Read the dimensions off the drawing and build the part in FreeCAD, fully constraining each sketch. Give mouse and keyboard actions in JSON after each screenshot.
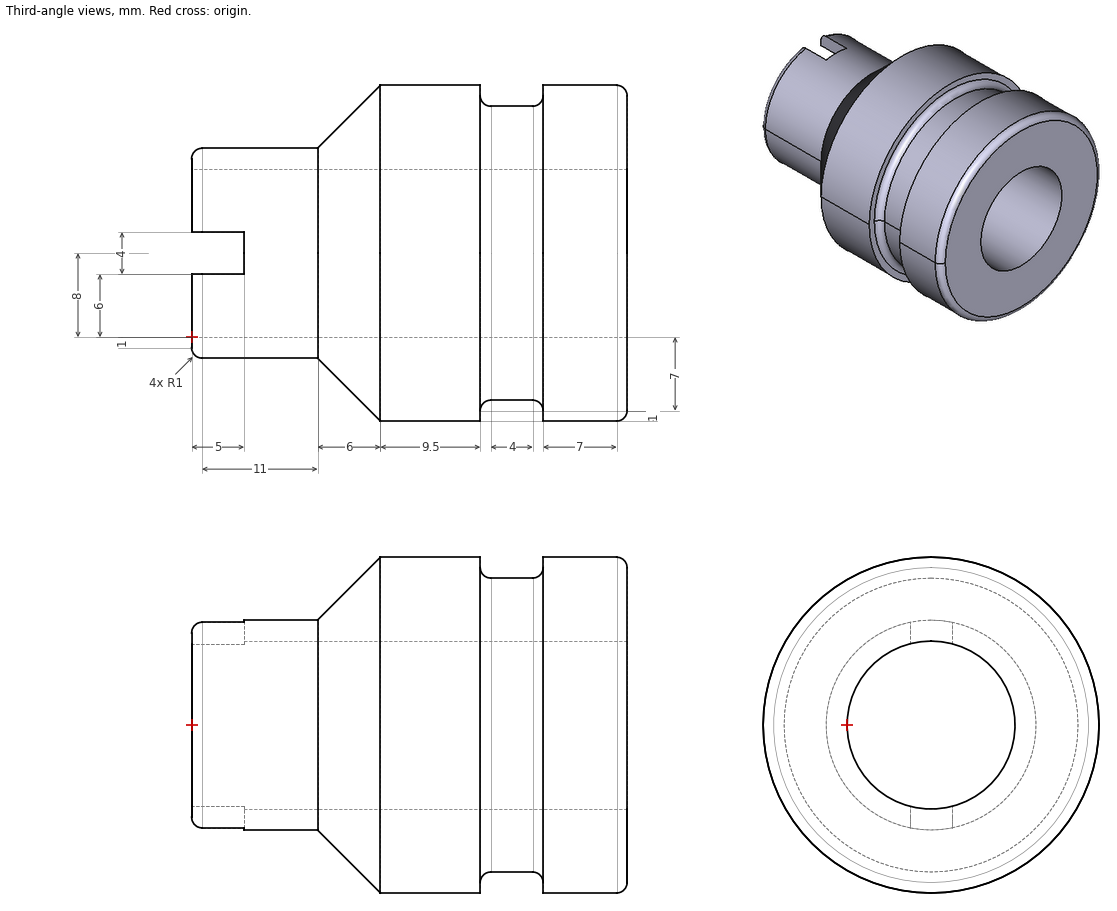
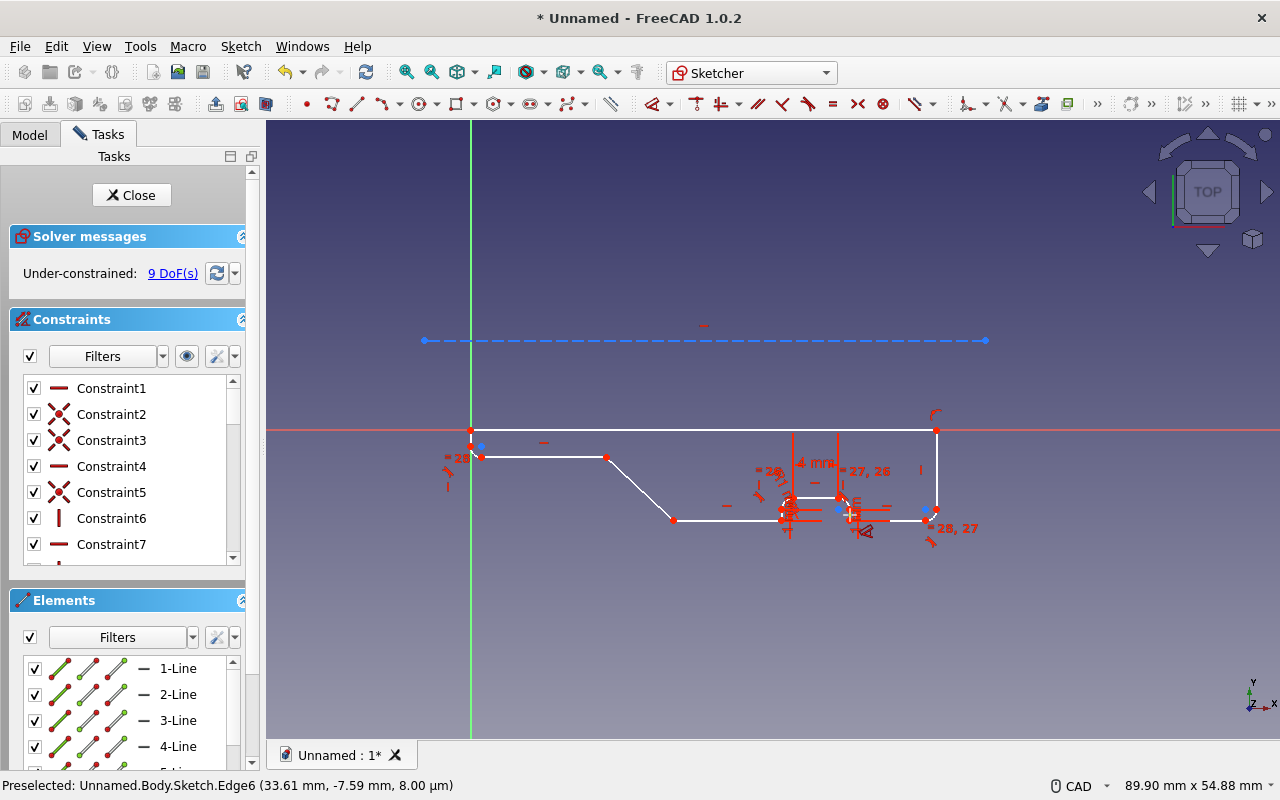
{"action": "left_click", "coordinate": [872, 521]}
{"action": "left_click", "coordinate": [888, 555]}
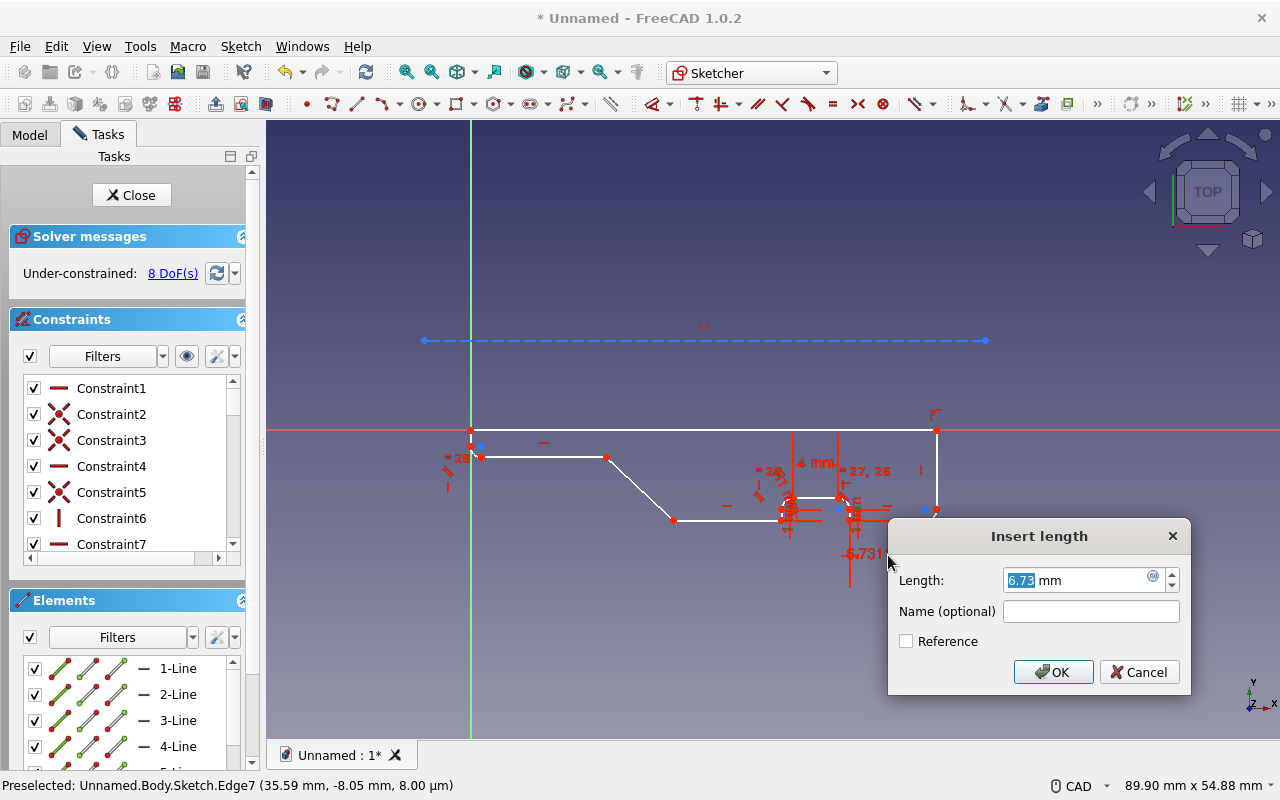
{"action": "type", "text": "7"}
{"action": "key", "text": "Return"}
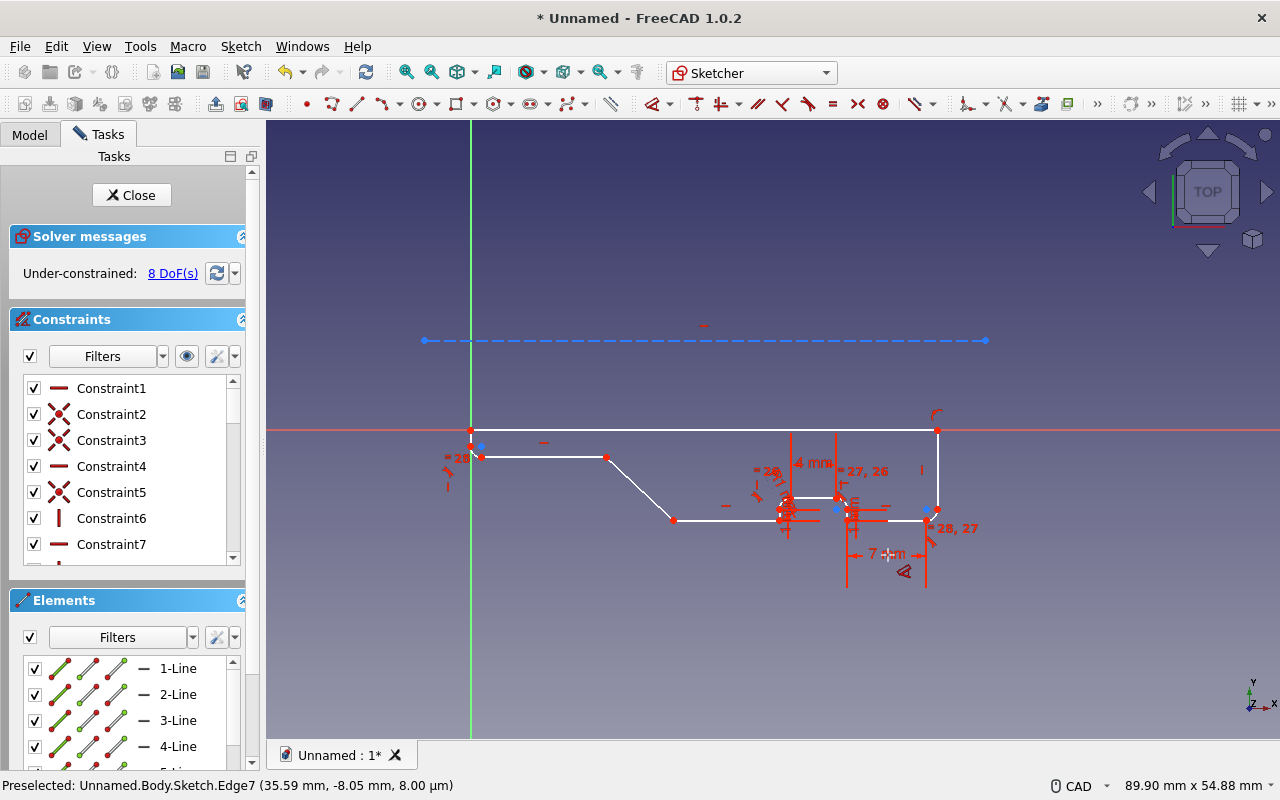
{"action": "left_click", "coordinate": [938, 486]}
{"action": "left_click", "coordinate": [972, 470]}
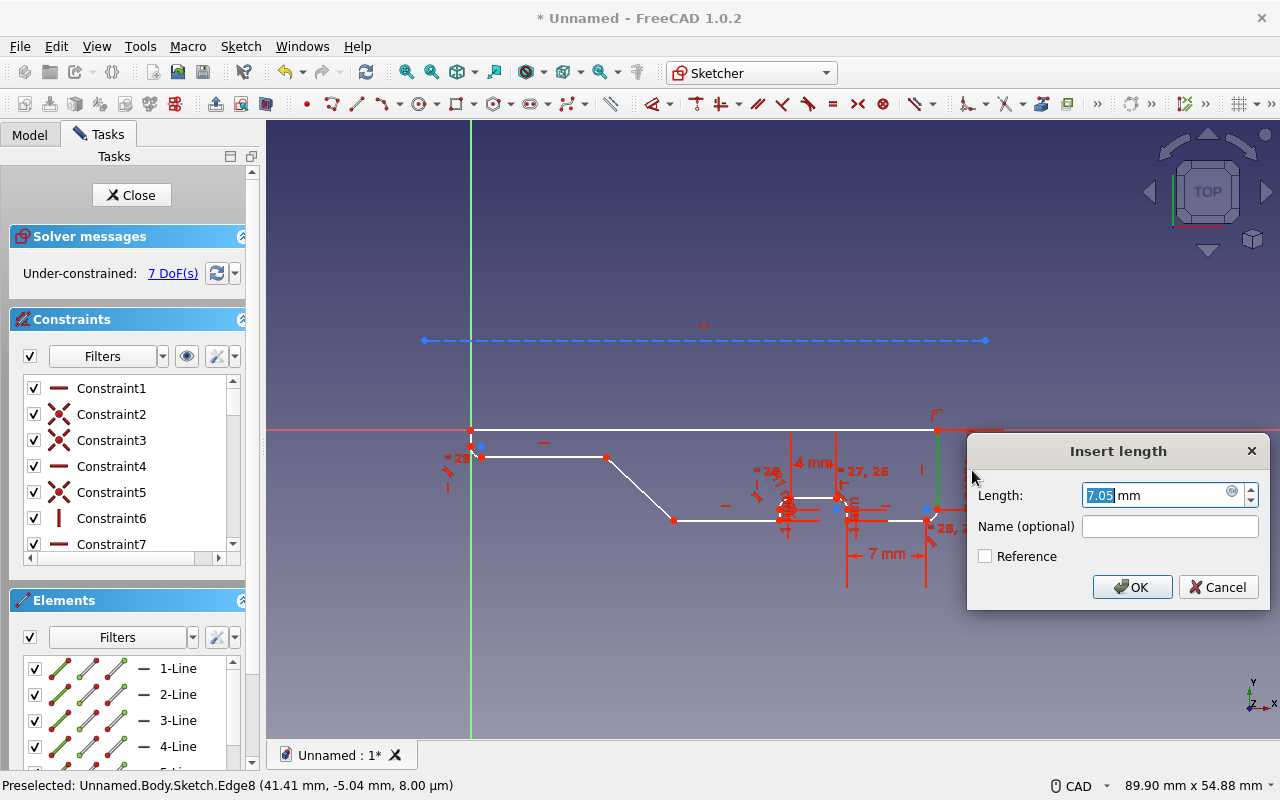
{"action": "type", "text": "7"}
{"action": "key", "text": "Return"}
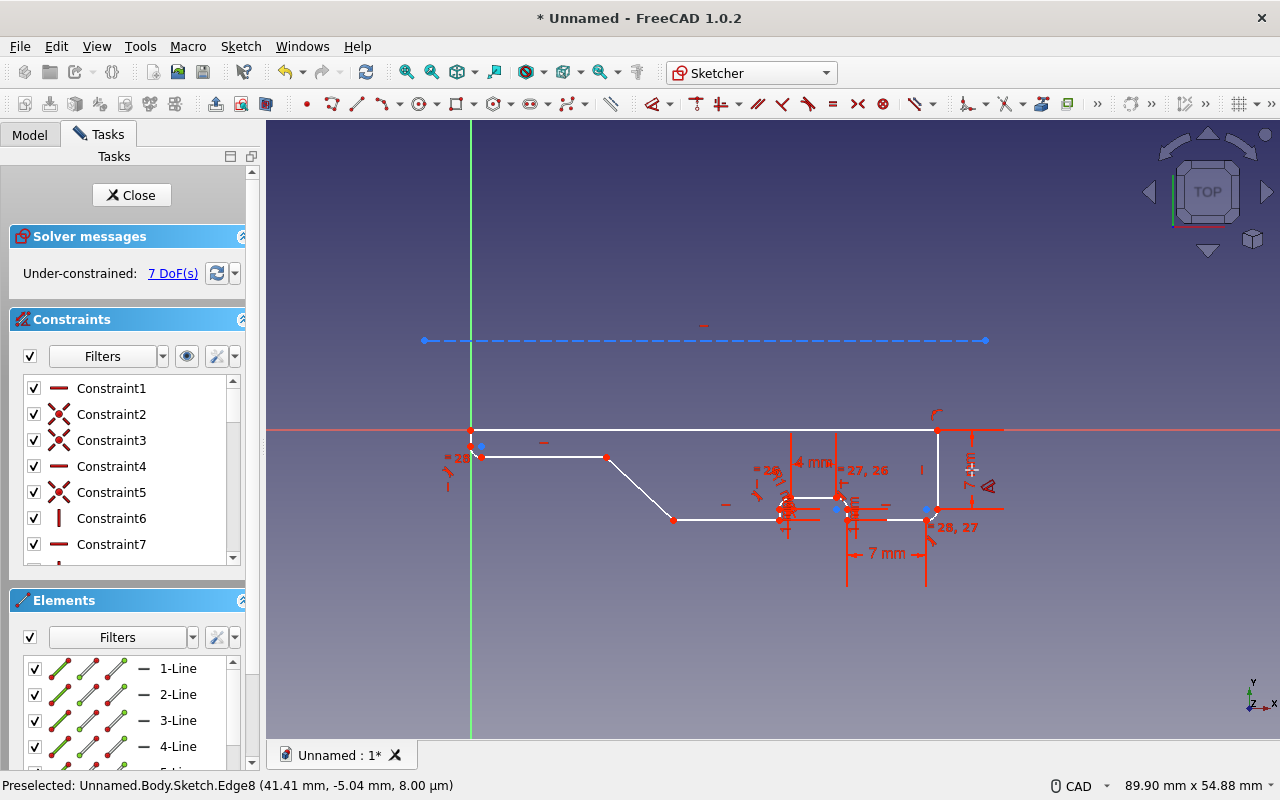
{"action": "scroll", "coordinate": [471, 438], "scroll_direction": "up", "scroll_amount": 7}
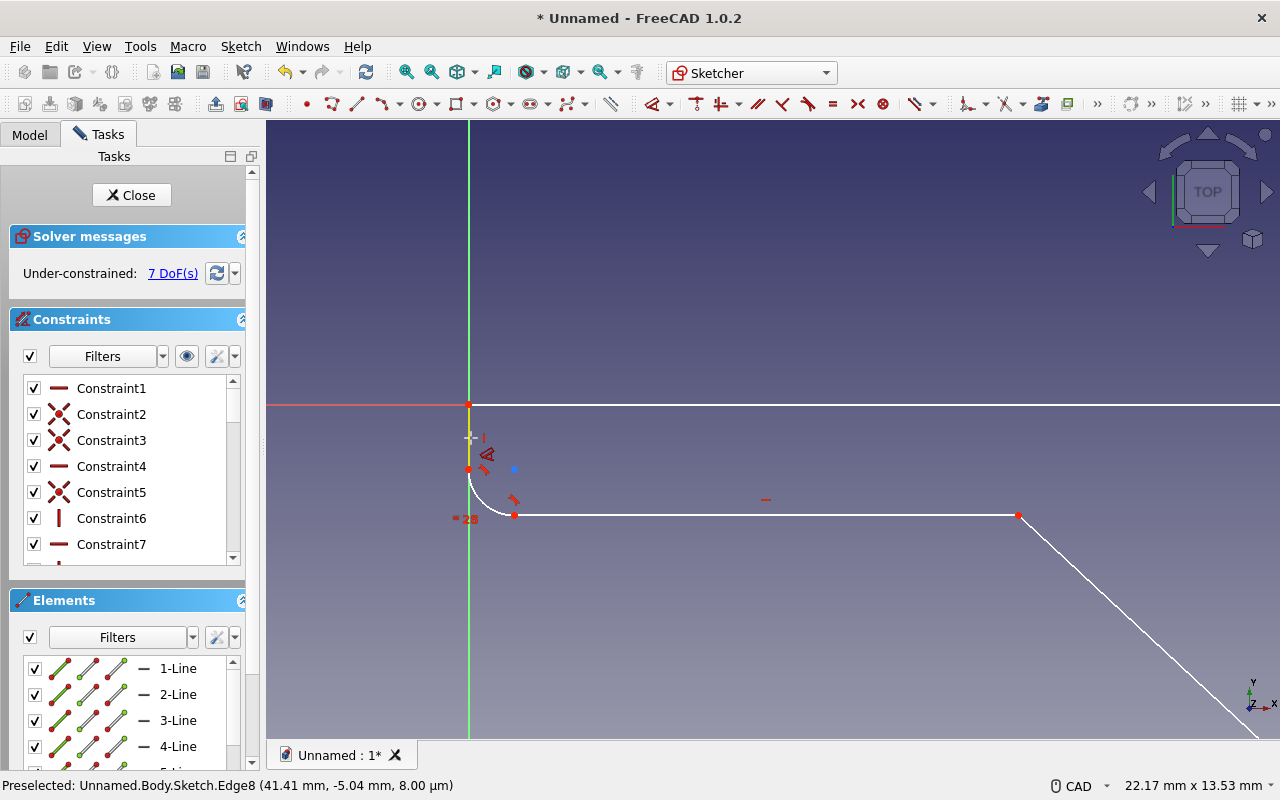
{"action": "left_click", "coordinate": [469, 437]}
{"action": "left_click", "coordinate": [435, 437]}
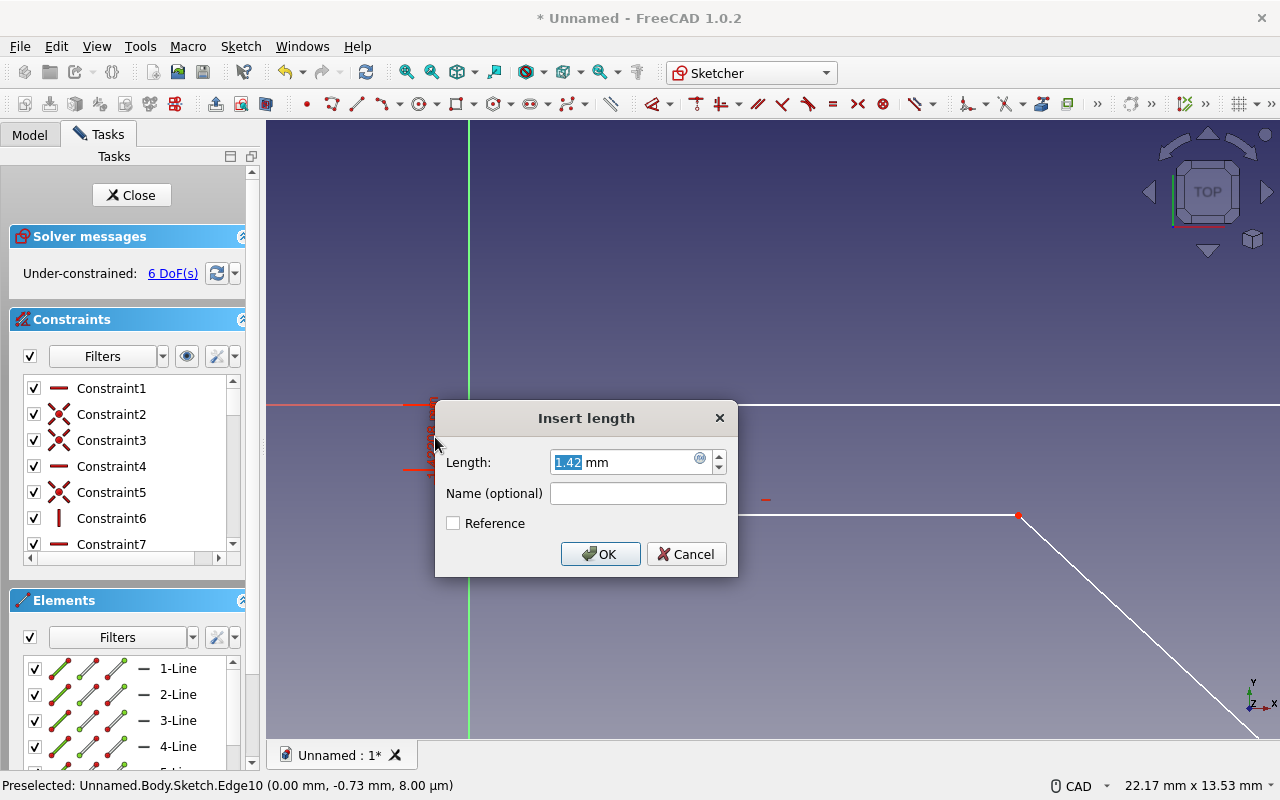
{"action": "type", "text": "1"}
{"action": "key", "text": "Return"}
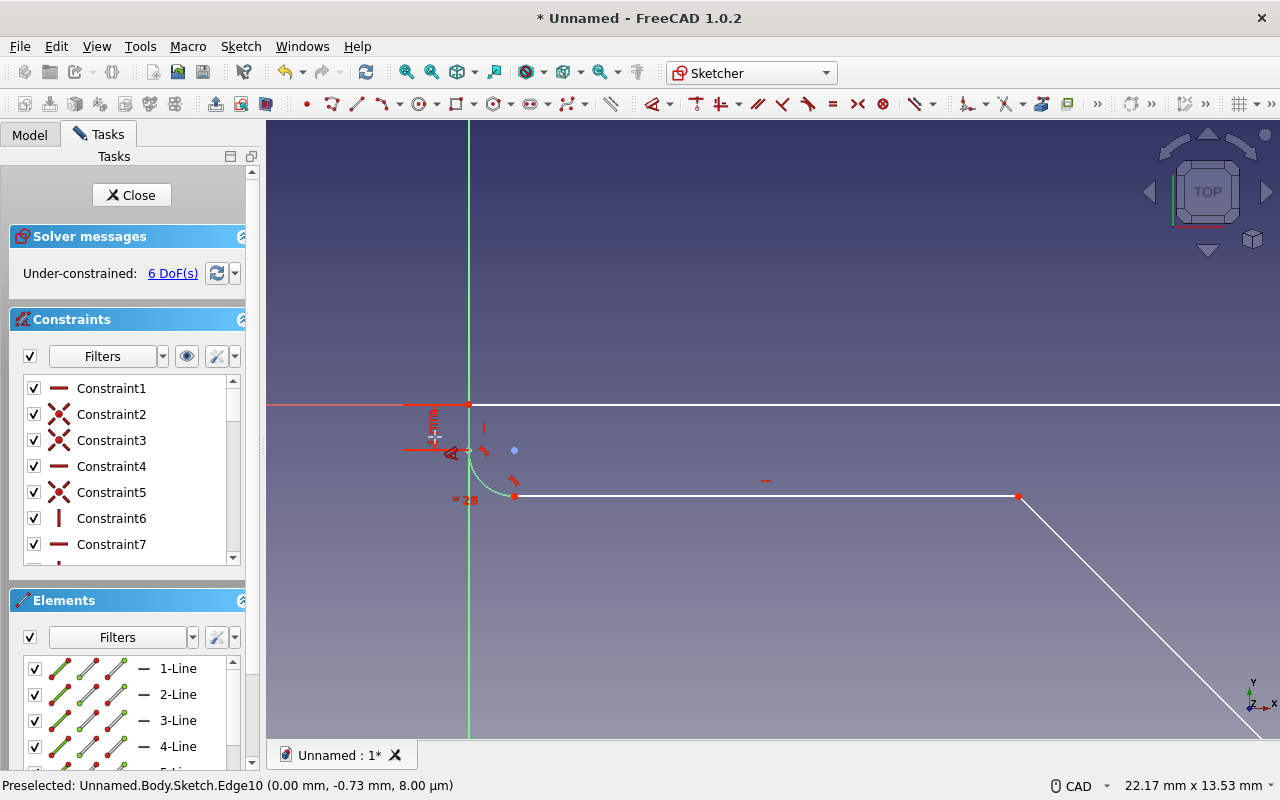
{"action": "scroll", "coordinate": [471, 438], "scroll_direction": "down", "scroll_amount": 7}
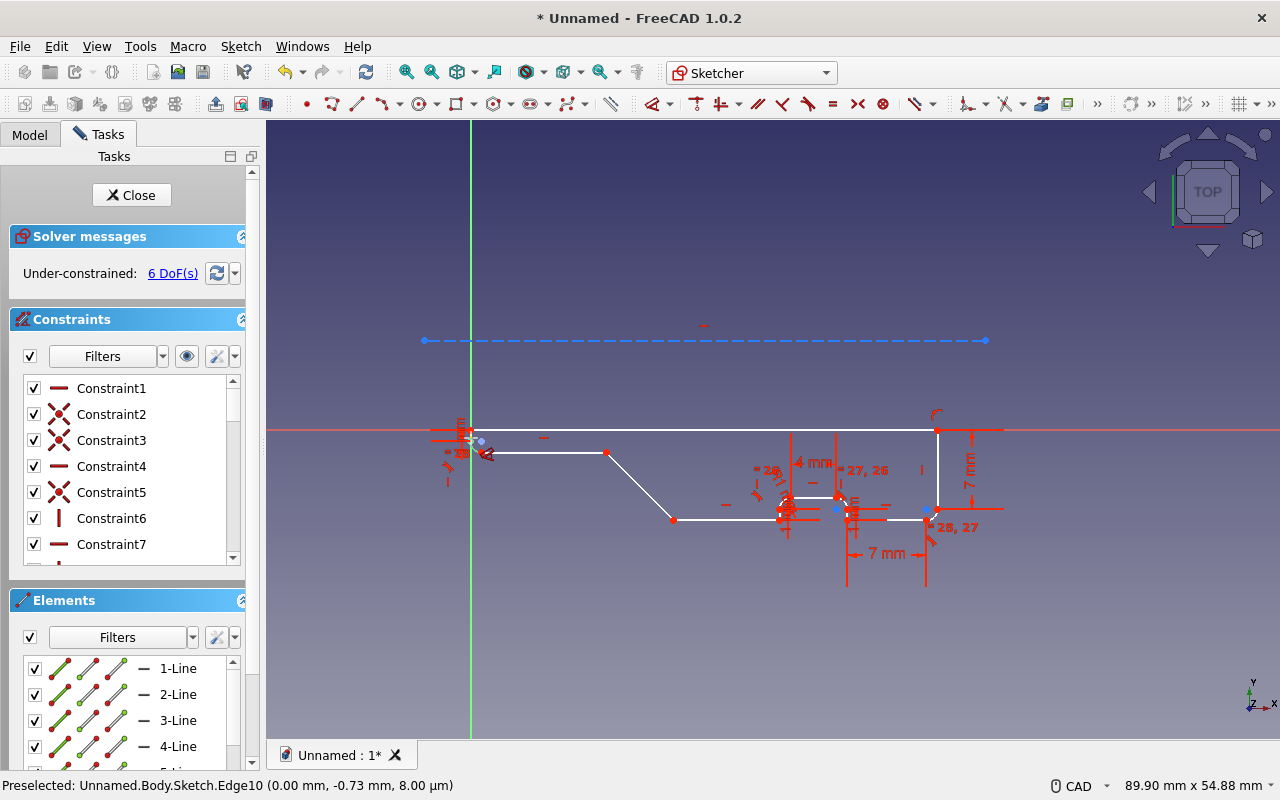
{"action": "left_click", "coordinate": [519, 453]}
{"action": "left_click", "coordinate": [544, 487]}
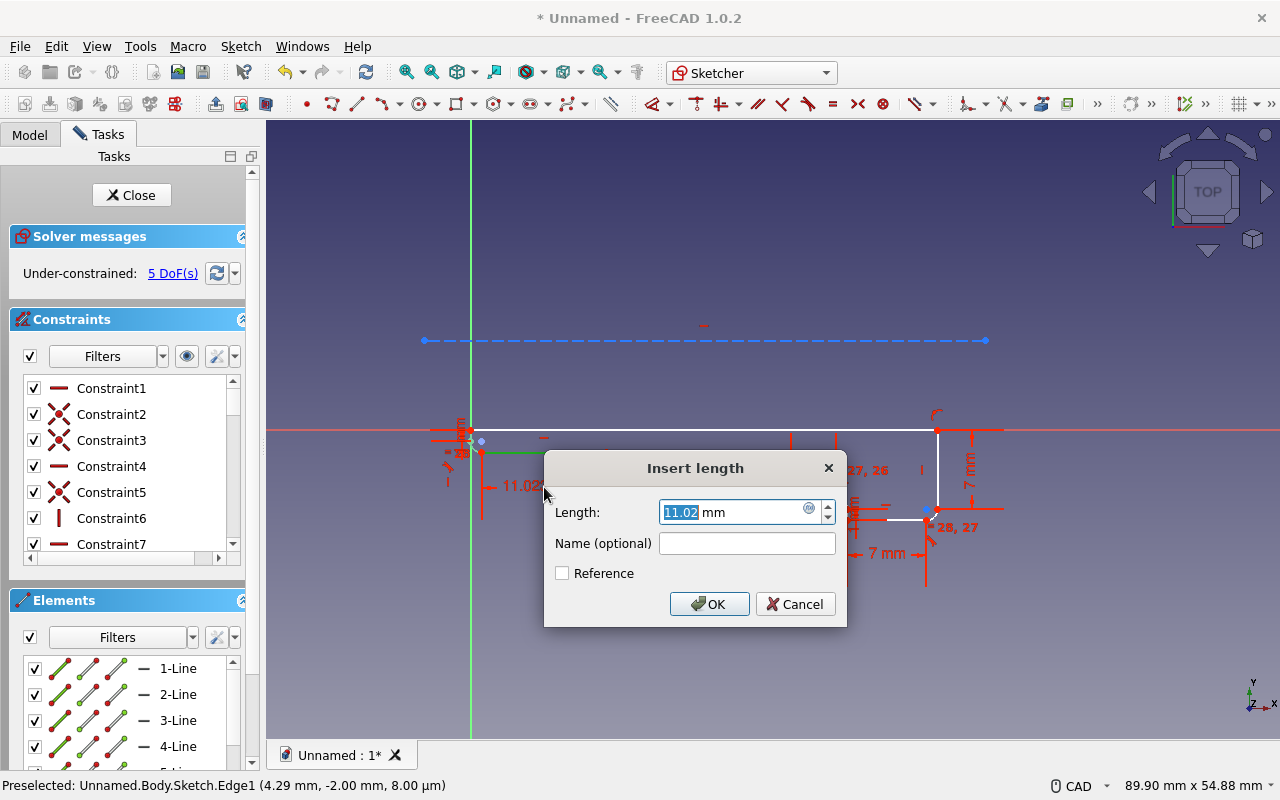
{"action": "type", "text": "11"}
{"action": "key", "text": "Return"}